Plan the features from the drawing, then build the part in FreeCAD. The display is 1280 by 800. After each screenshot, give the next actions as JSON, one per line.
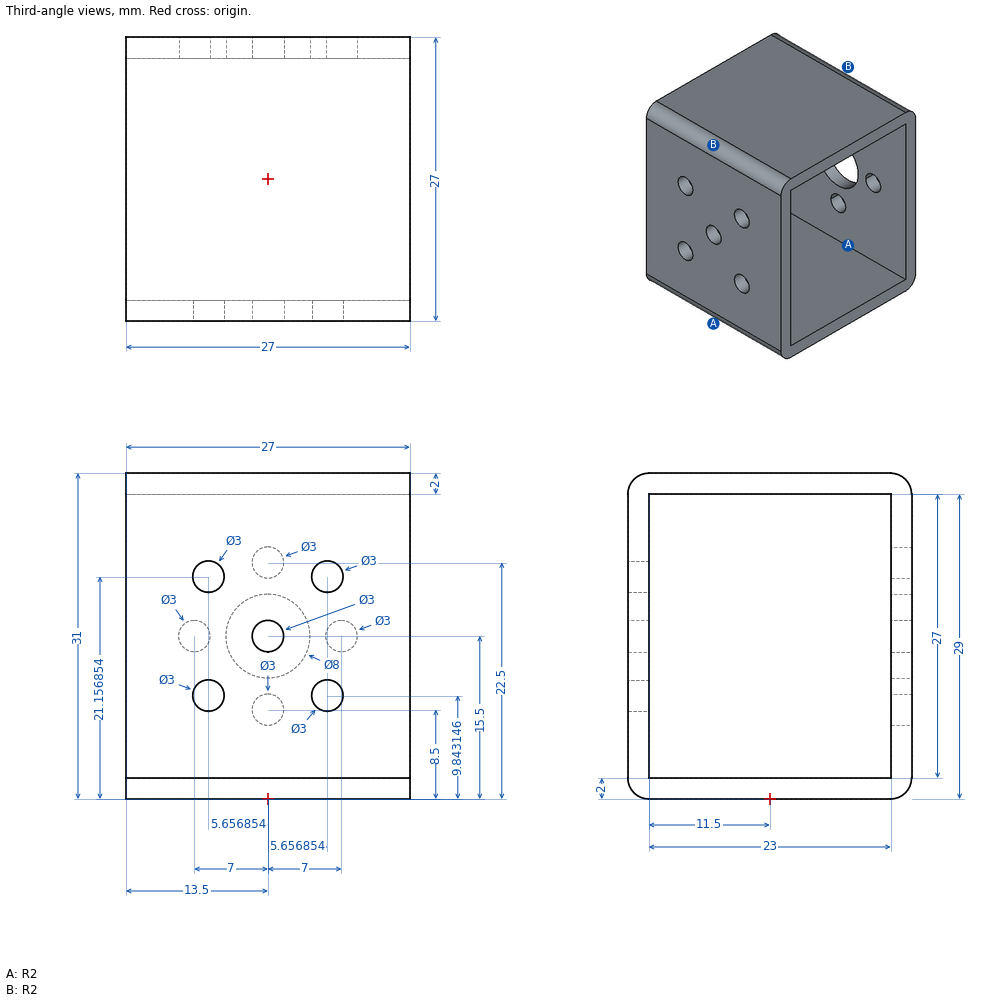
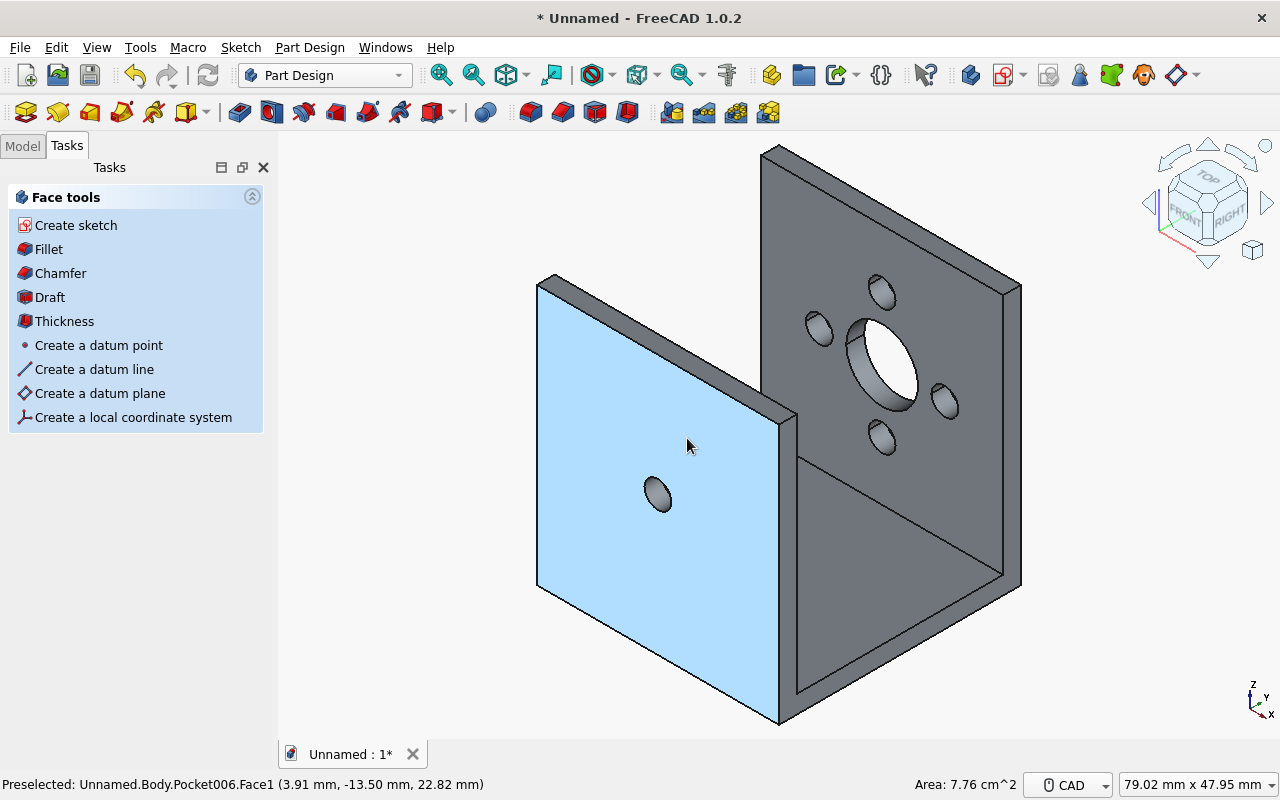
{"action": "left_click", "coordinate": [1004, 76]}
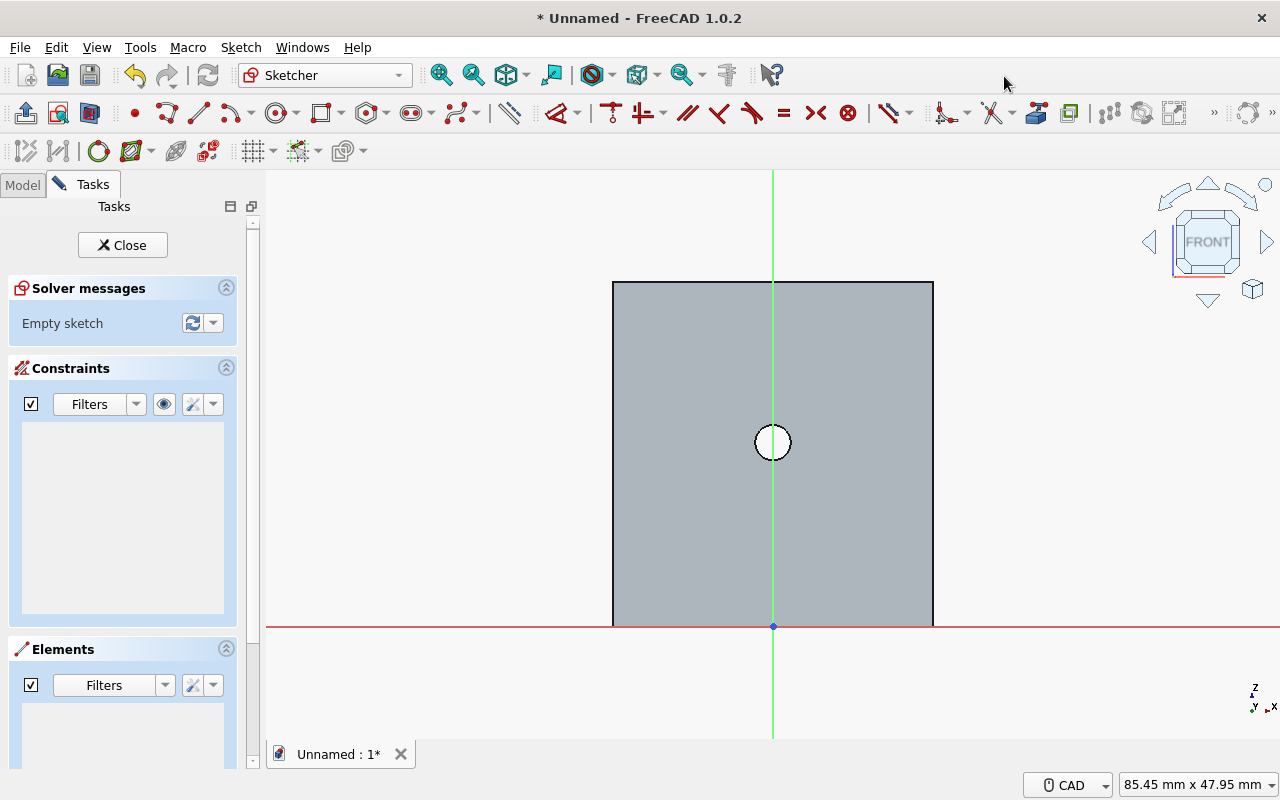
{"action": "scroll", "coordinate": [706, 368], "scroll_direction": "up", "scroll_amount": 12}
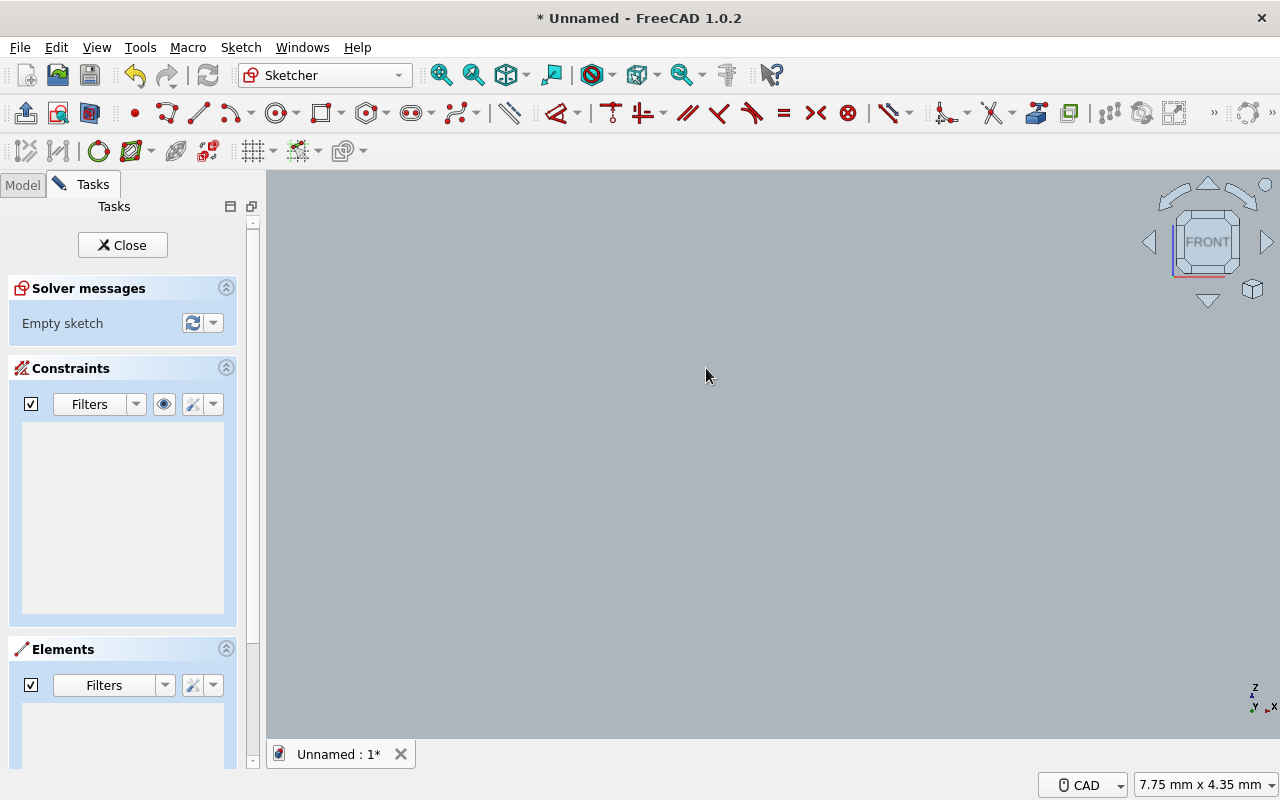
{"action": "key", "text": "g c"}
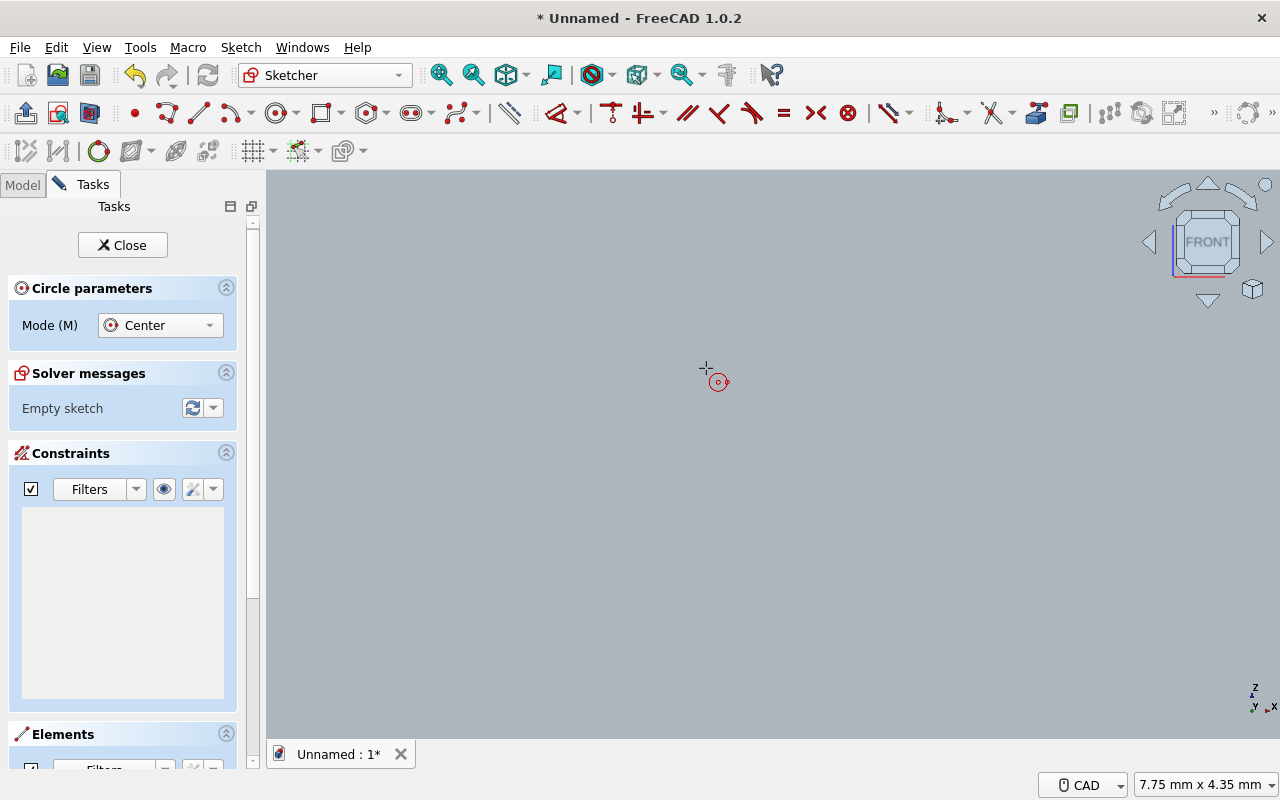
{"action": "left_click", "coordinate": [700, 447]}
{"action": "mouse_move", "coordinate": [839, 308]}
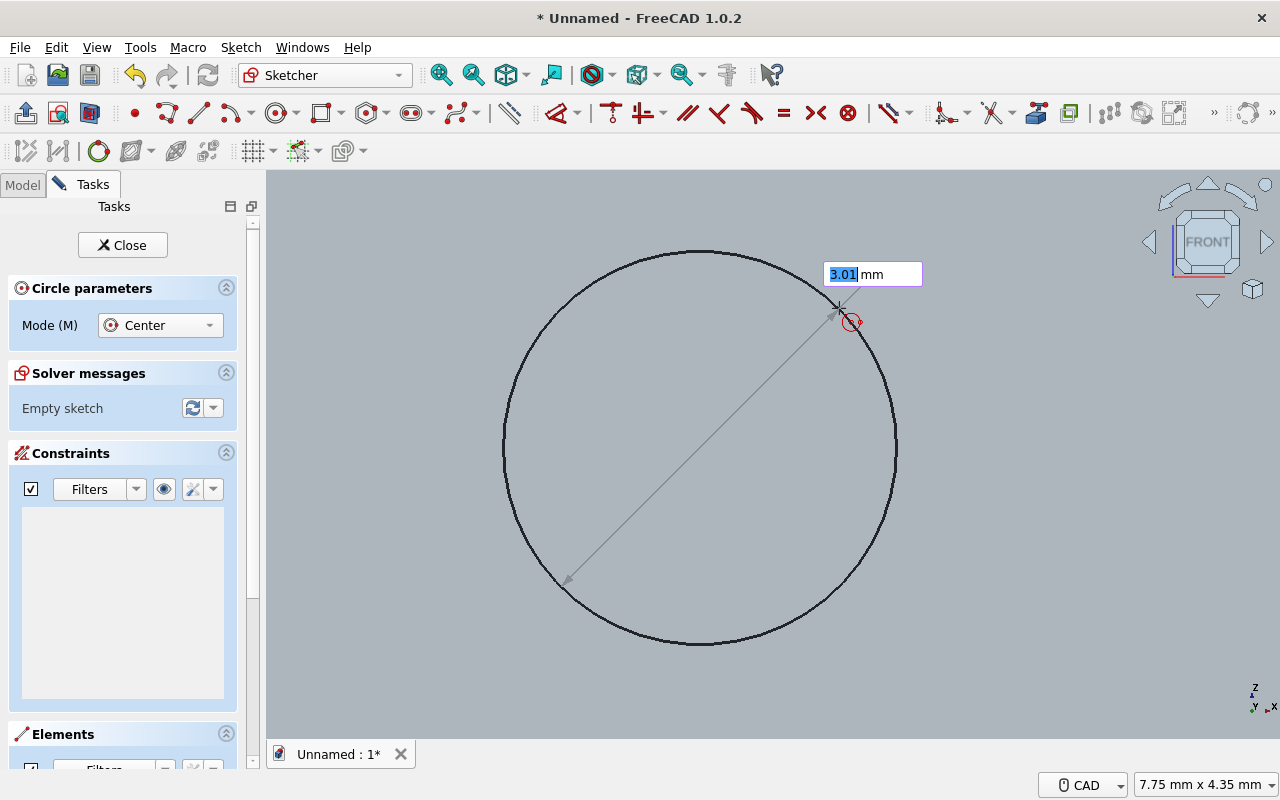
{"action": "type", "text": "3"}
{"action": "key", "text": "Return"}
{"action": "key", "text": "Escape"}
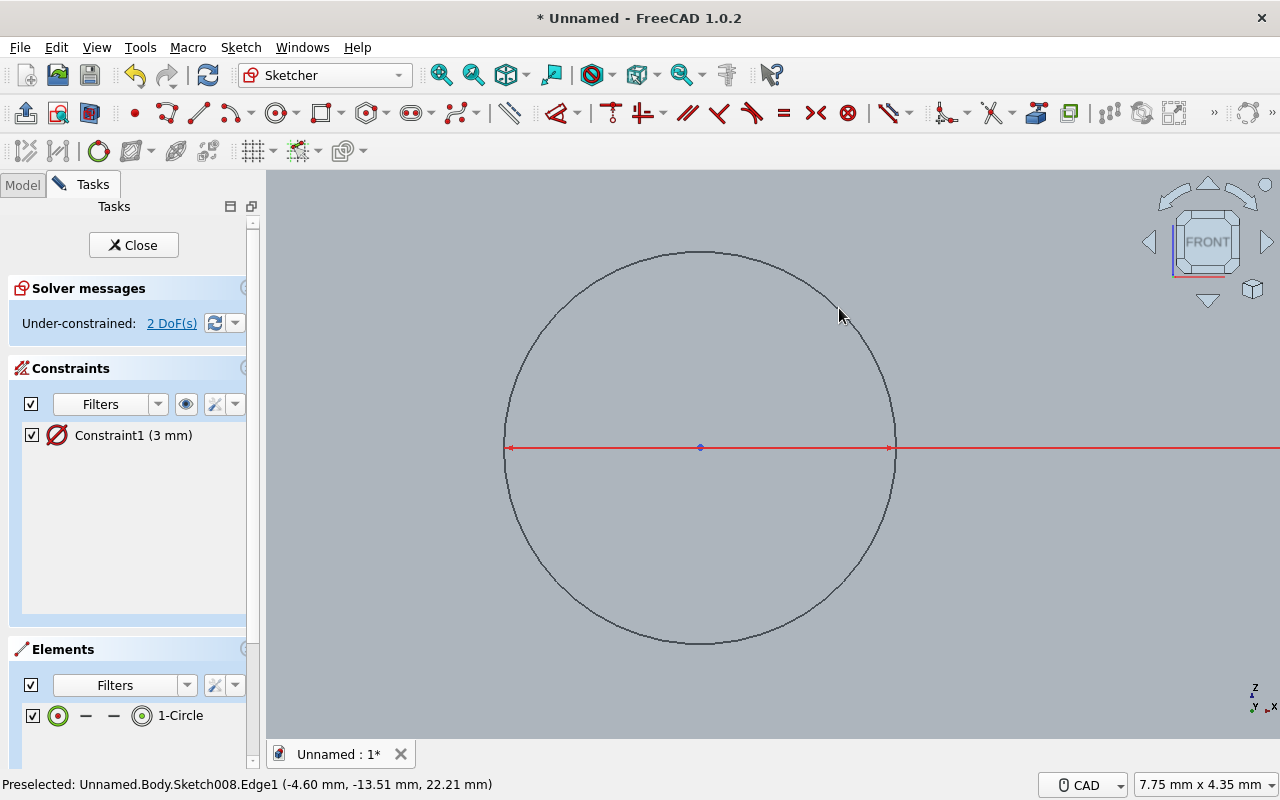
{"action": "left_click", "coordinate": [556, 114]}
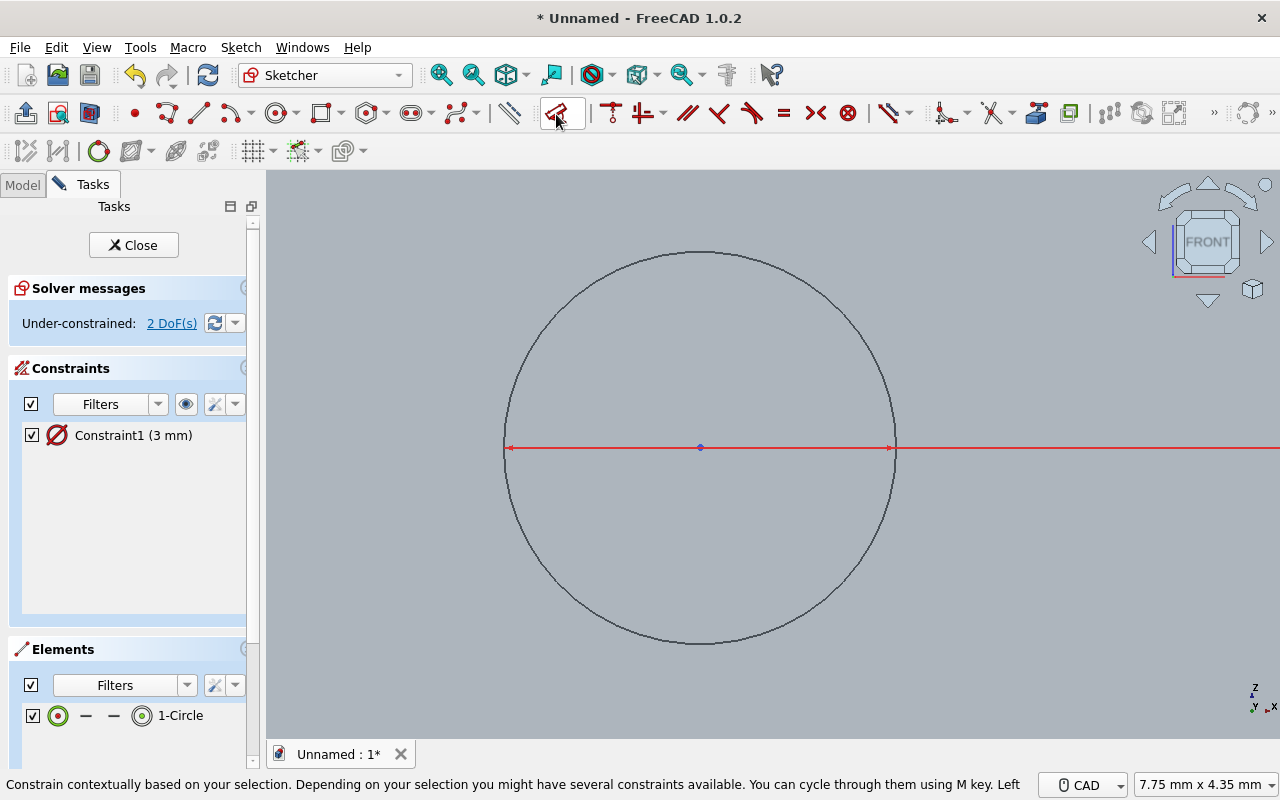
{"action": "left_click", "coordinate": [700, 448]}
{"action": "left_click", "coordinate": [907, 414]}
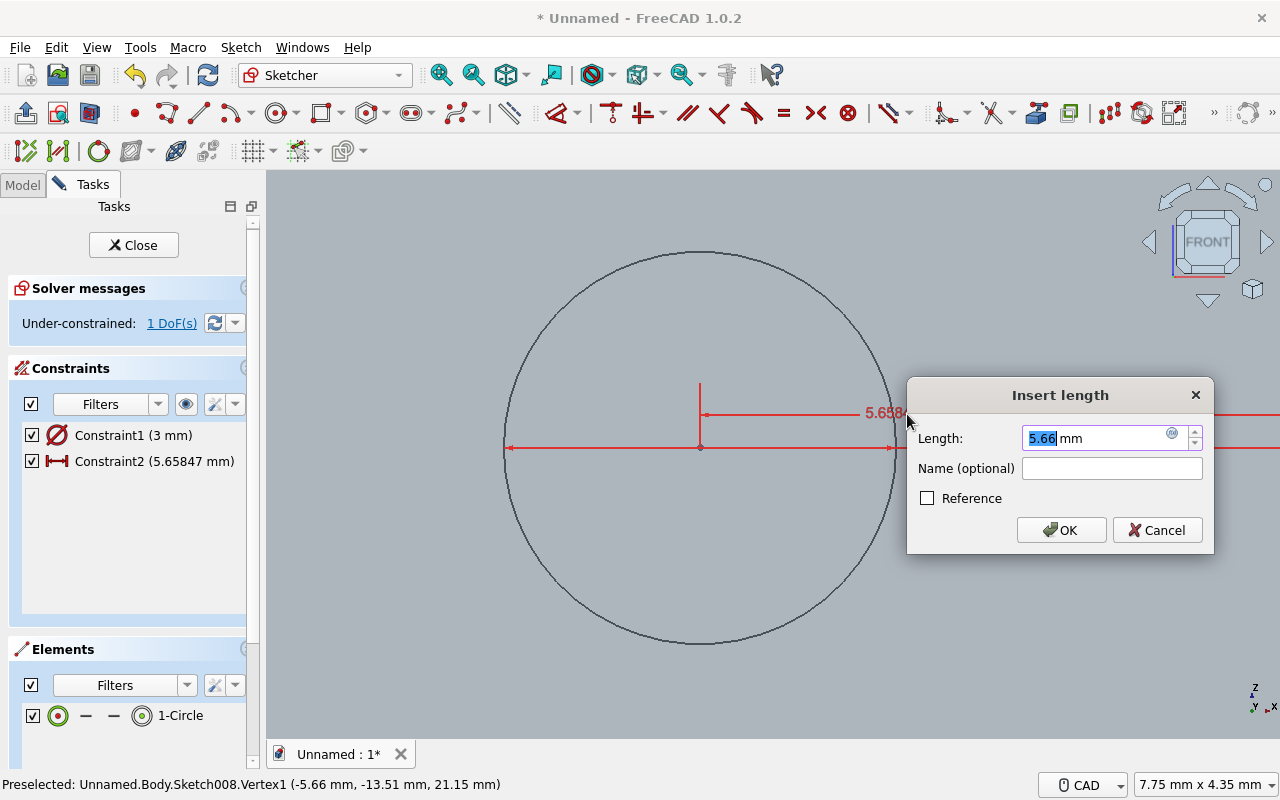
{"action": "type", "text": "5.656854"}
{"action": "key", "text": "Return"}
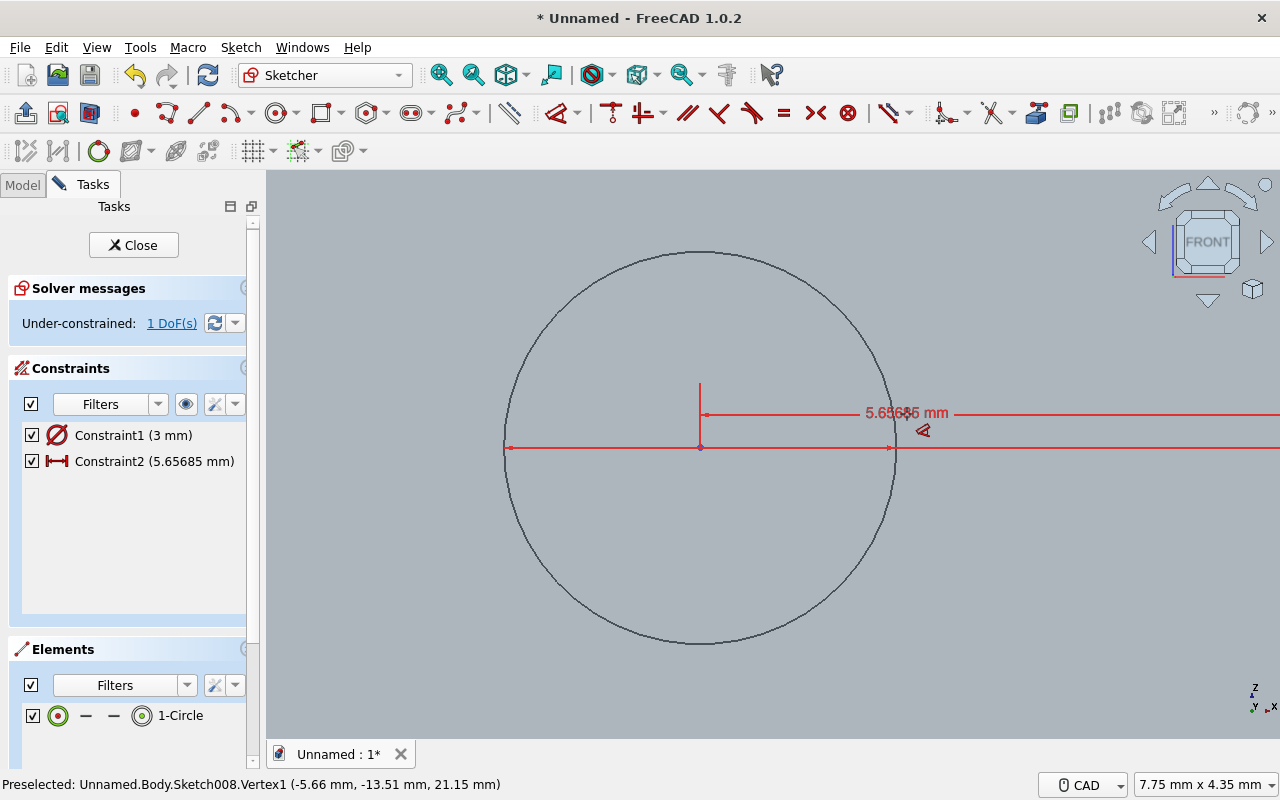
{"action": "left_click", "coordinate": [700, 448]}
{"action": "left_click", "coordinate": [666, 579]}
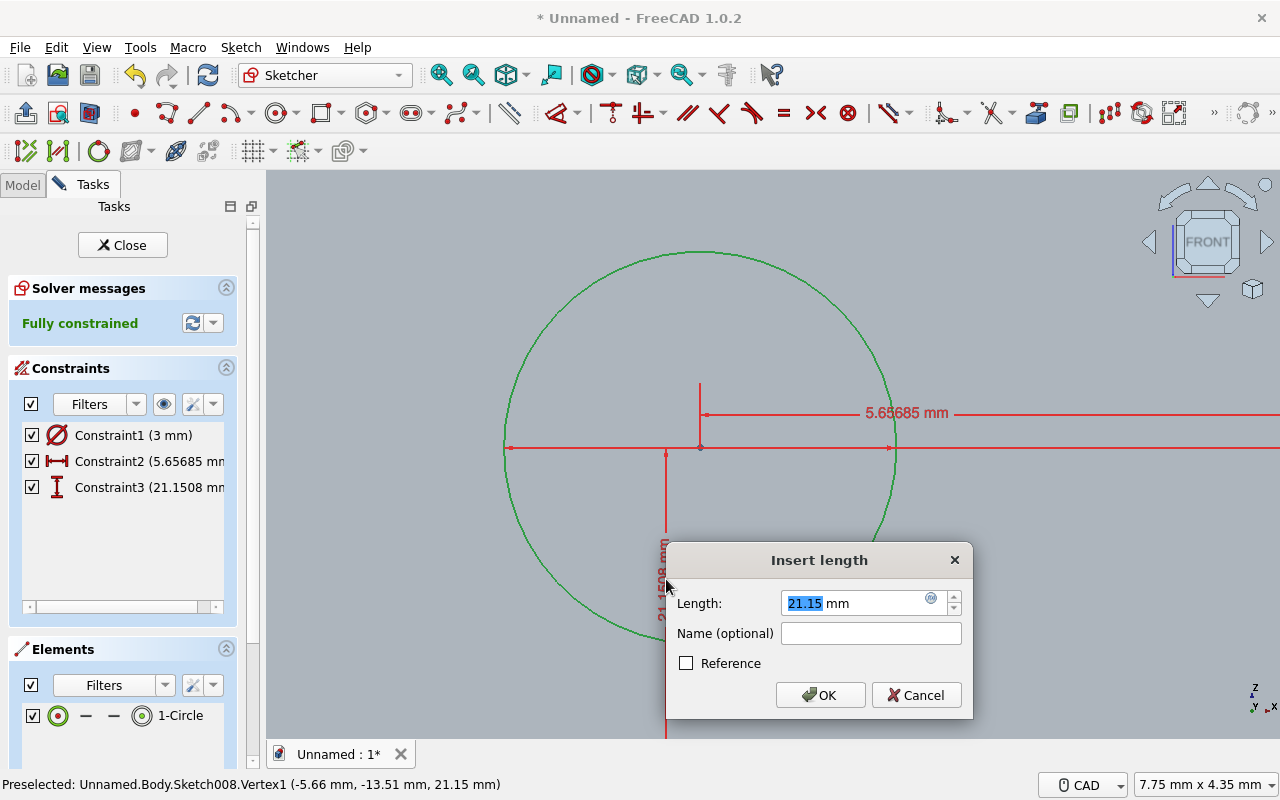
{"action": "type", "text": "21.156854"}
{"action": "key", "text": "Return"}
{"action": "key", "text": "Escape"}